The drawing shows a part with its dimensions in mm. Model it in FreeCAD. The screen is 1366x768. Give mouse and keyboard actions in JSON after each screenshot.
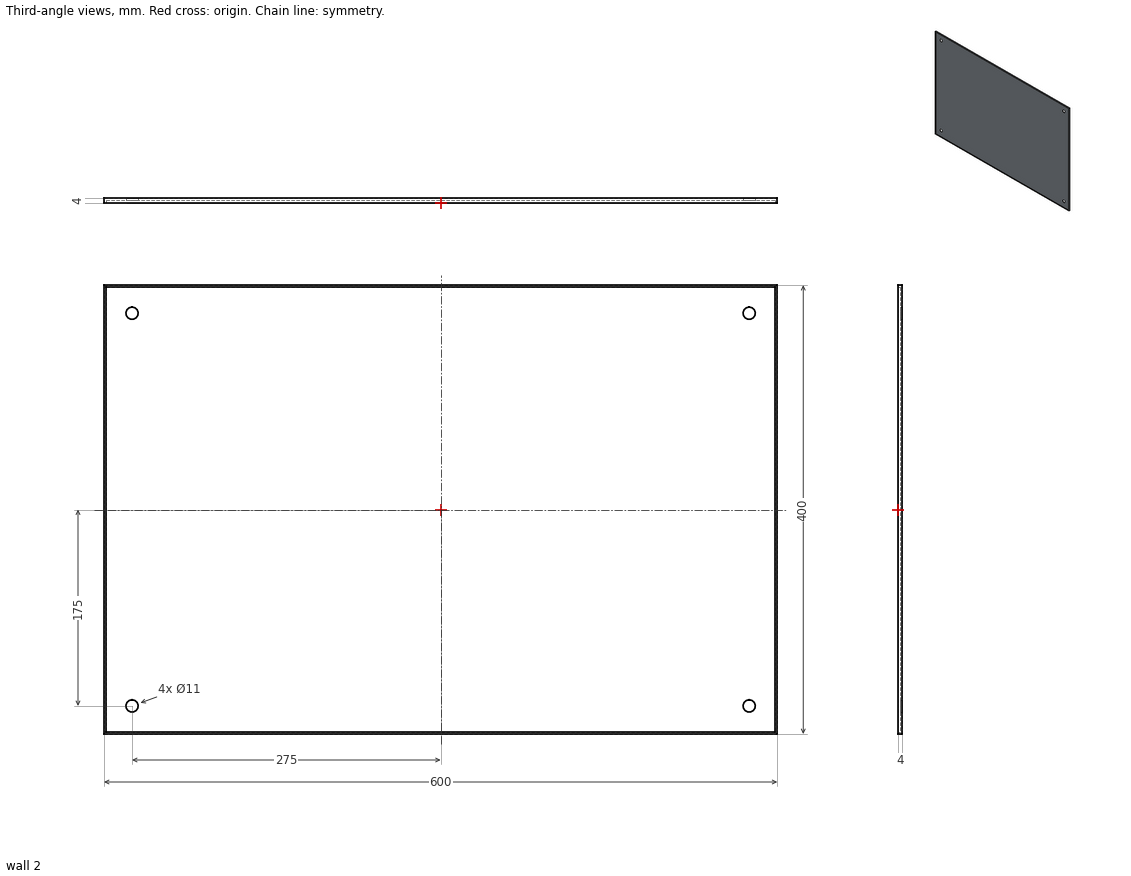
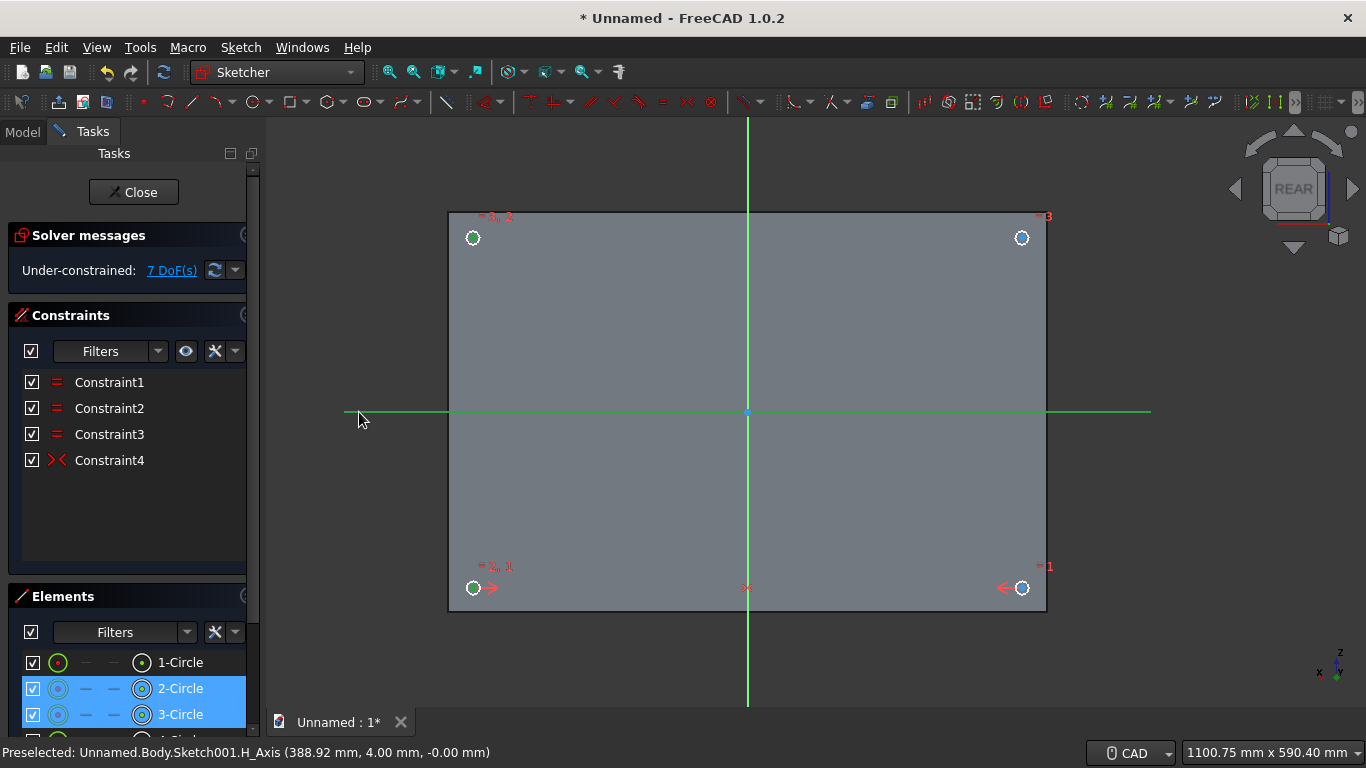
{"action": "key", "text": "s"}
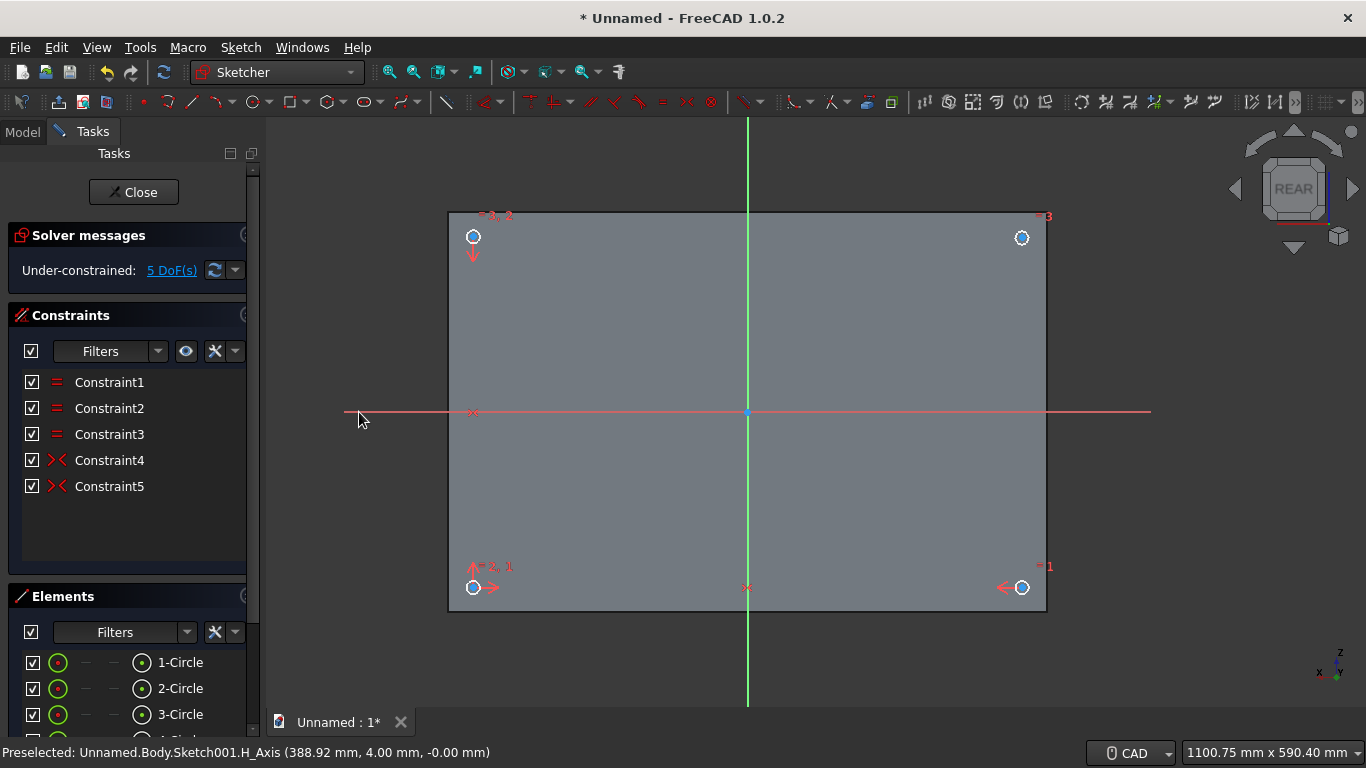
{"action": "left_click", "coordinate": [1022, 588]}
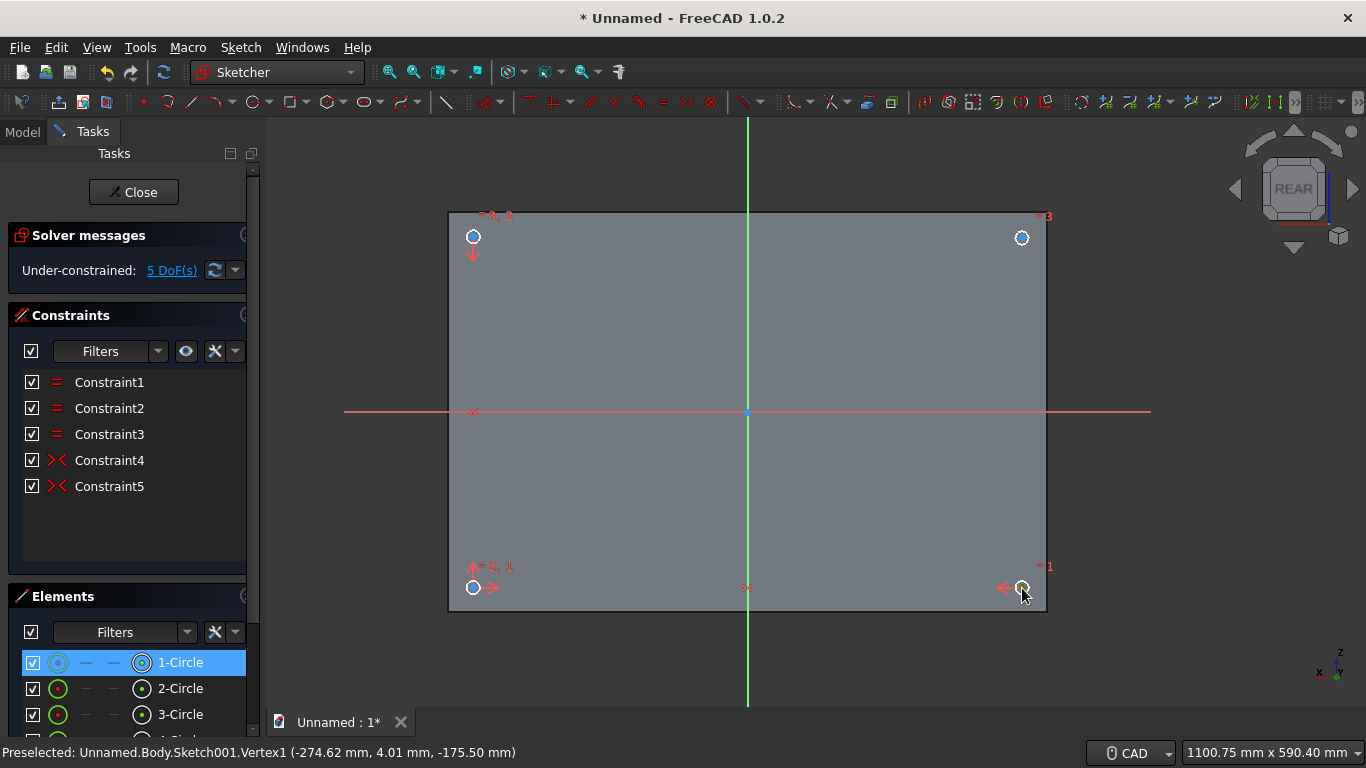
{"action": "left_click", "coordinate": [1022, 238]}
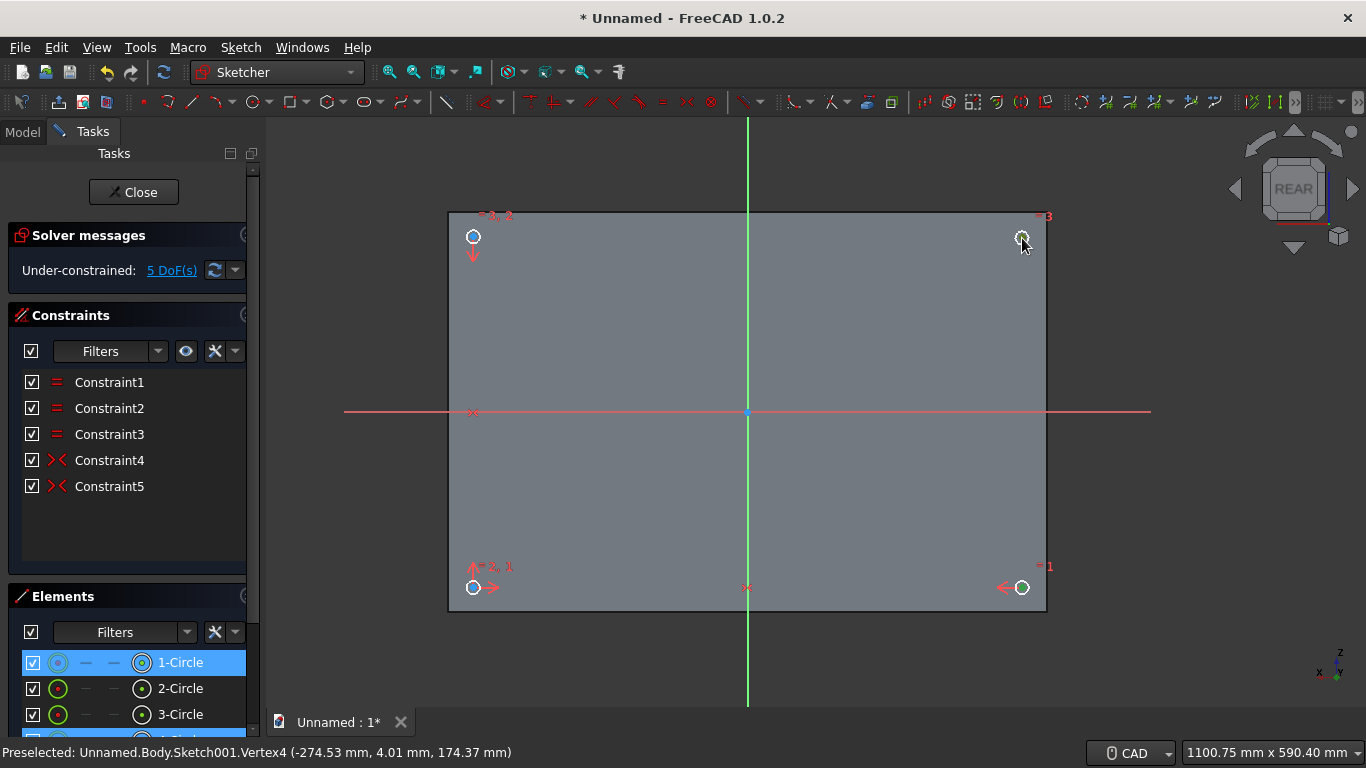
{"action": "left_click", "coordinate": [359, 412]}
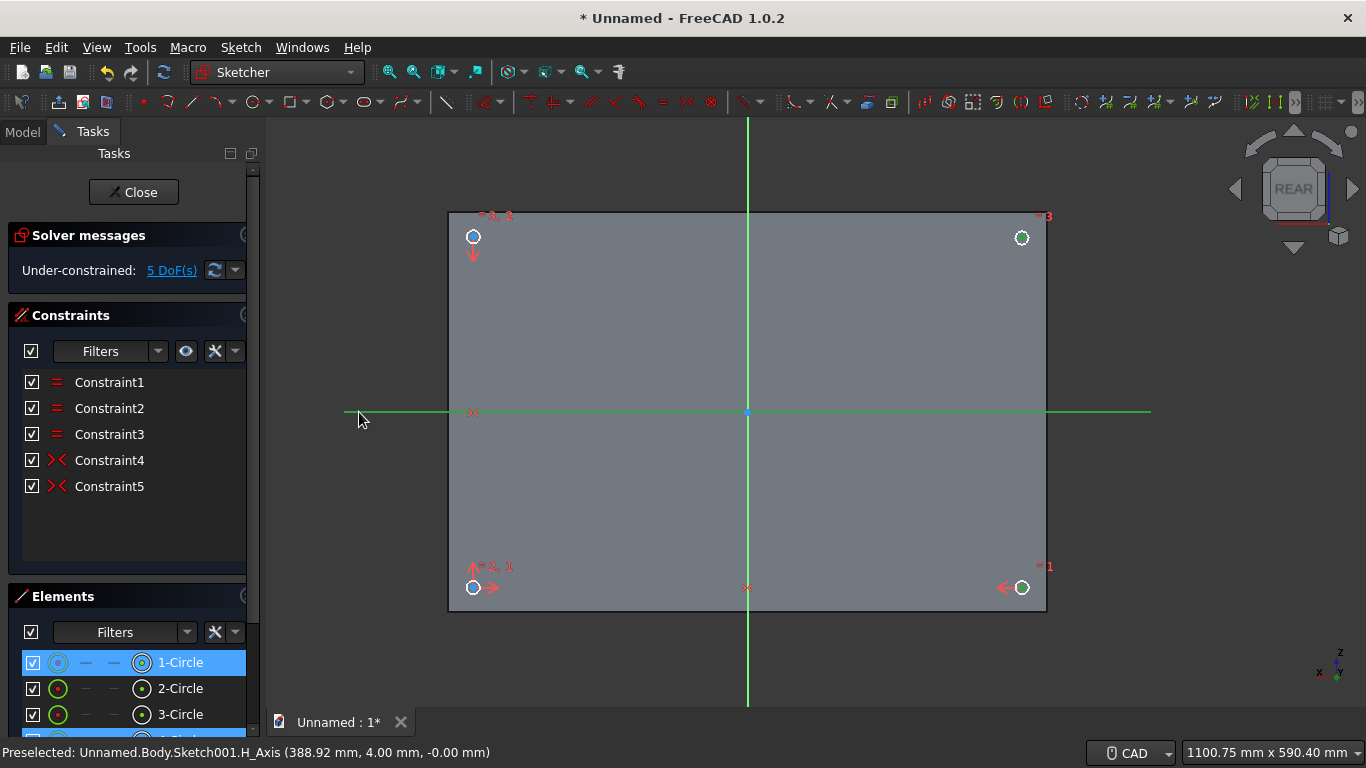
{"action": "left_click", "coordinate": [688, 102]}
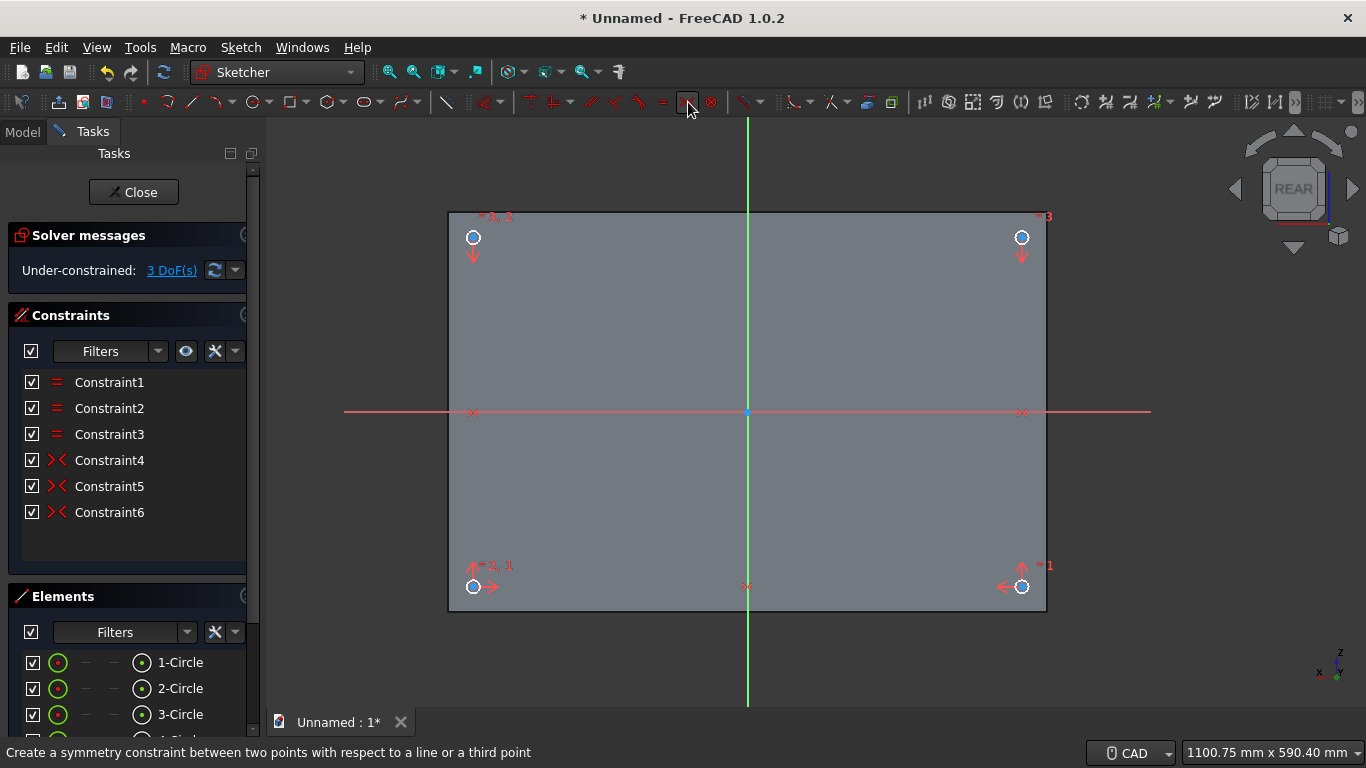
{"action": "key", "text": "d"}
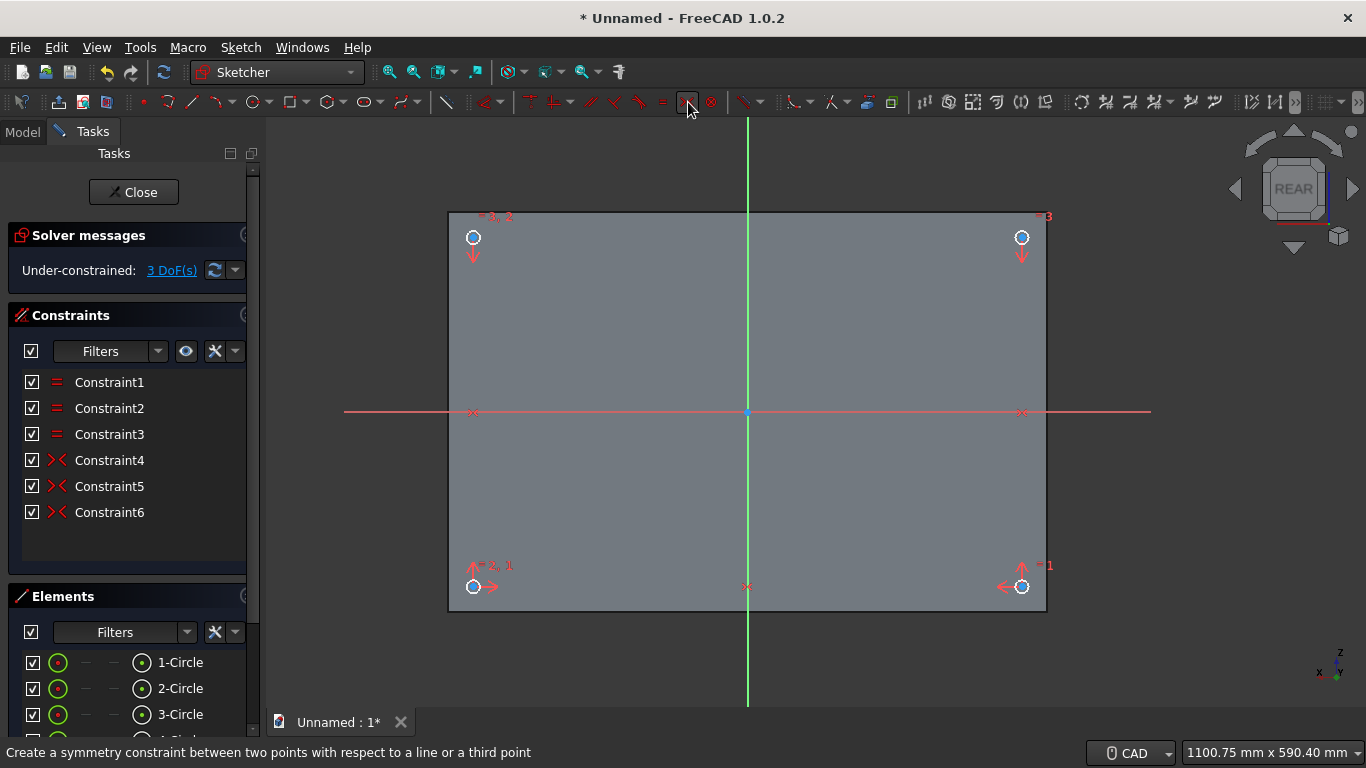
{"action": "scroll", "coordinate": [1022, 580], "scroll_direction": "up", "scroll_amount": 7}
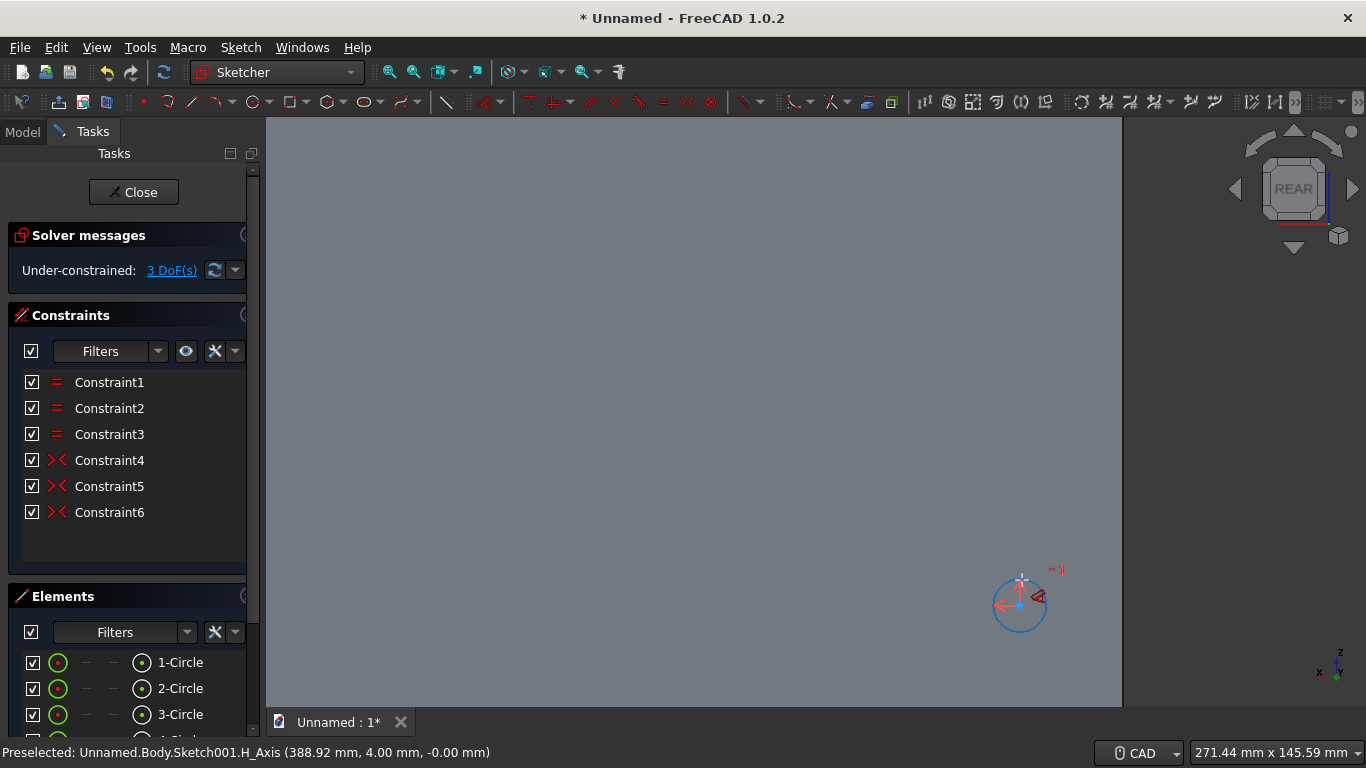
{"action": "left_click", "coordinate": [1021, 579]}
{"action": "left_click", "coordinate": [1022, 547]}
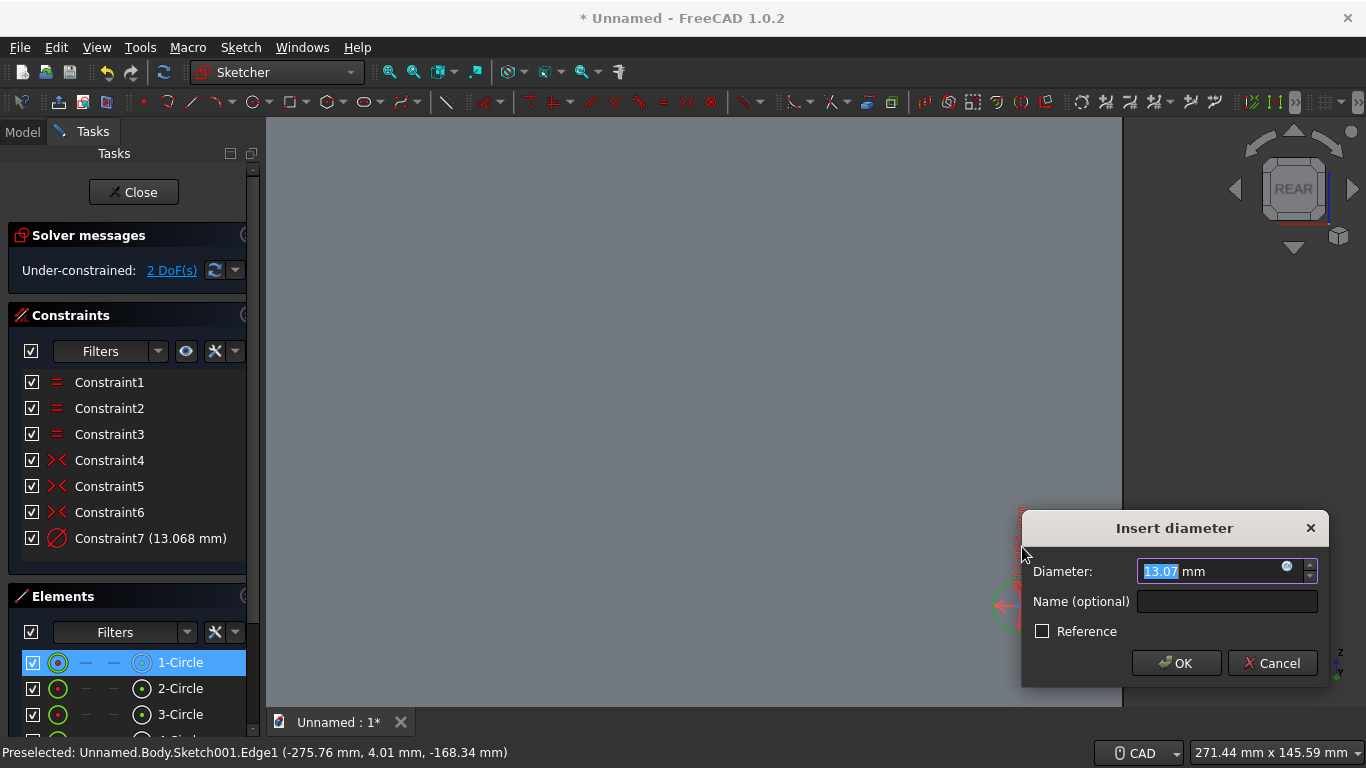
{"action": "type", "text": "11"}
{"action": "key", "text": "Return"}